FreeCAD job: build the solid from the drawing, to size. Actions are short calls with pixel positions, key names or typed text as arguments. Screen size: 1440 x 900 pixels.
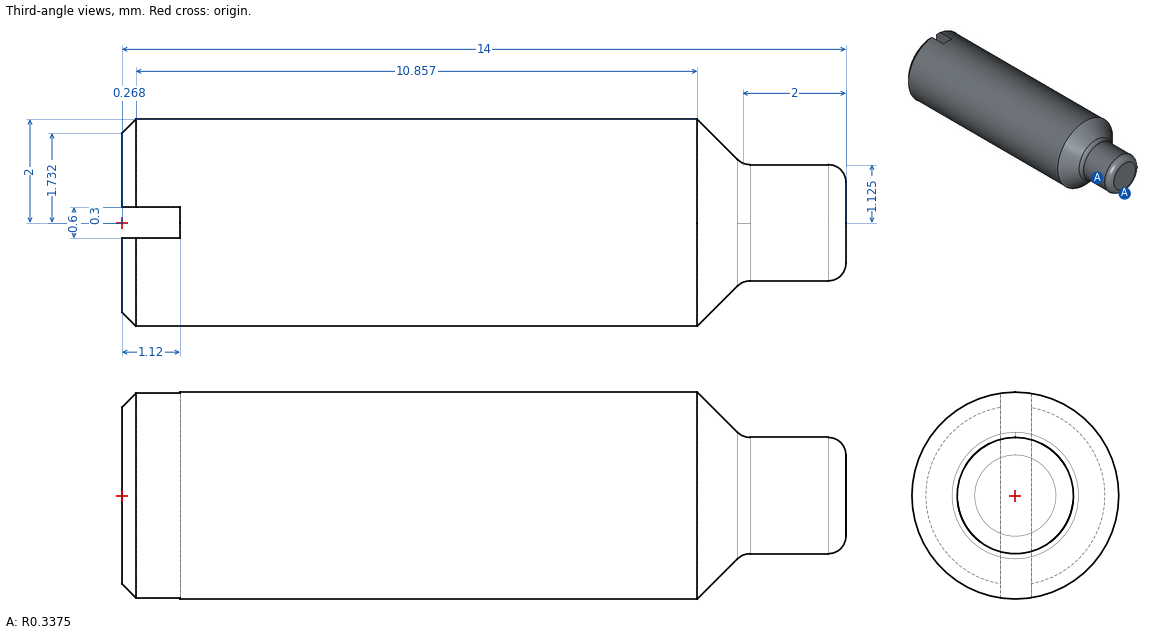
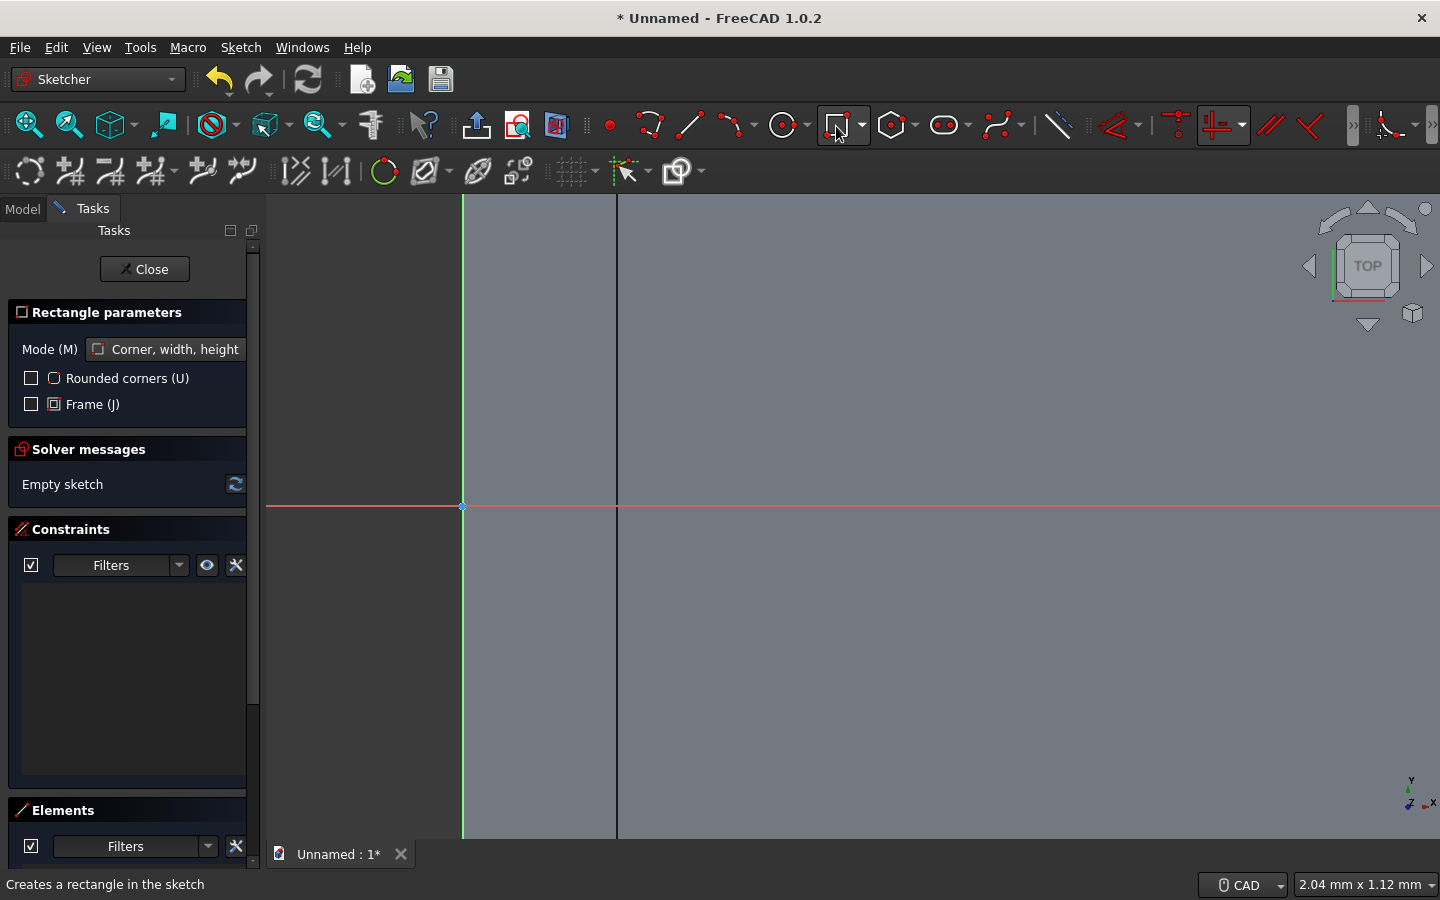
click(463, 334)
click(1107, 679)
key(Escape)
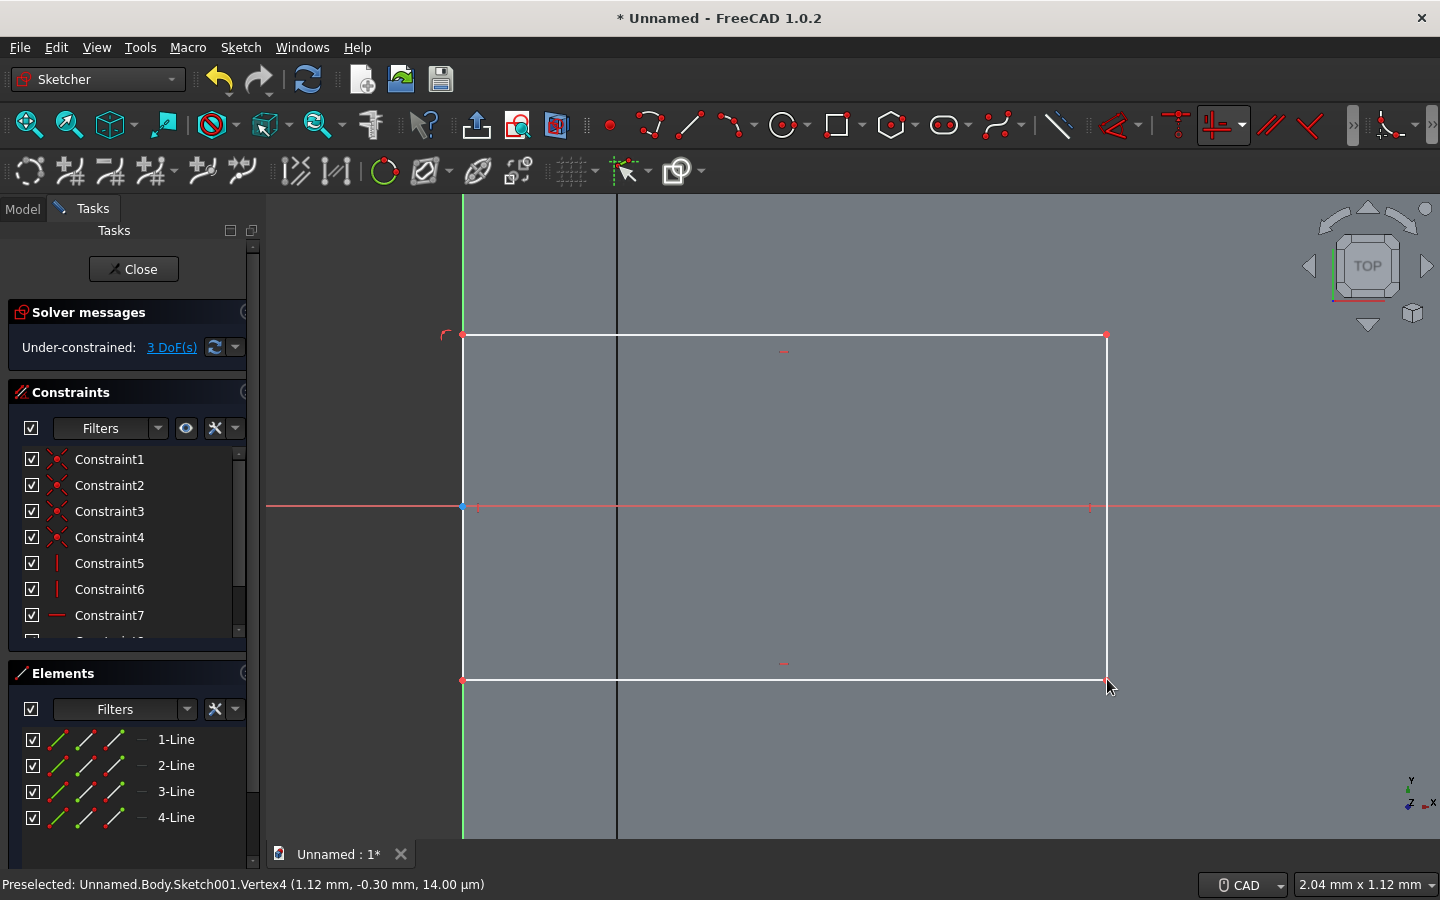
key(d)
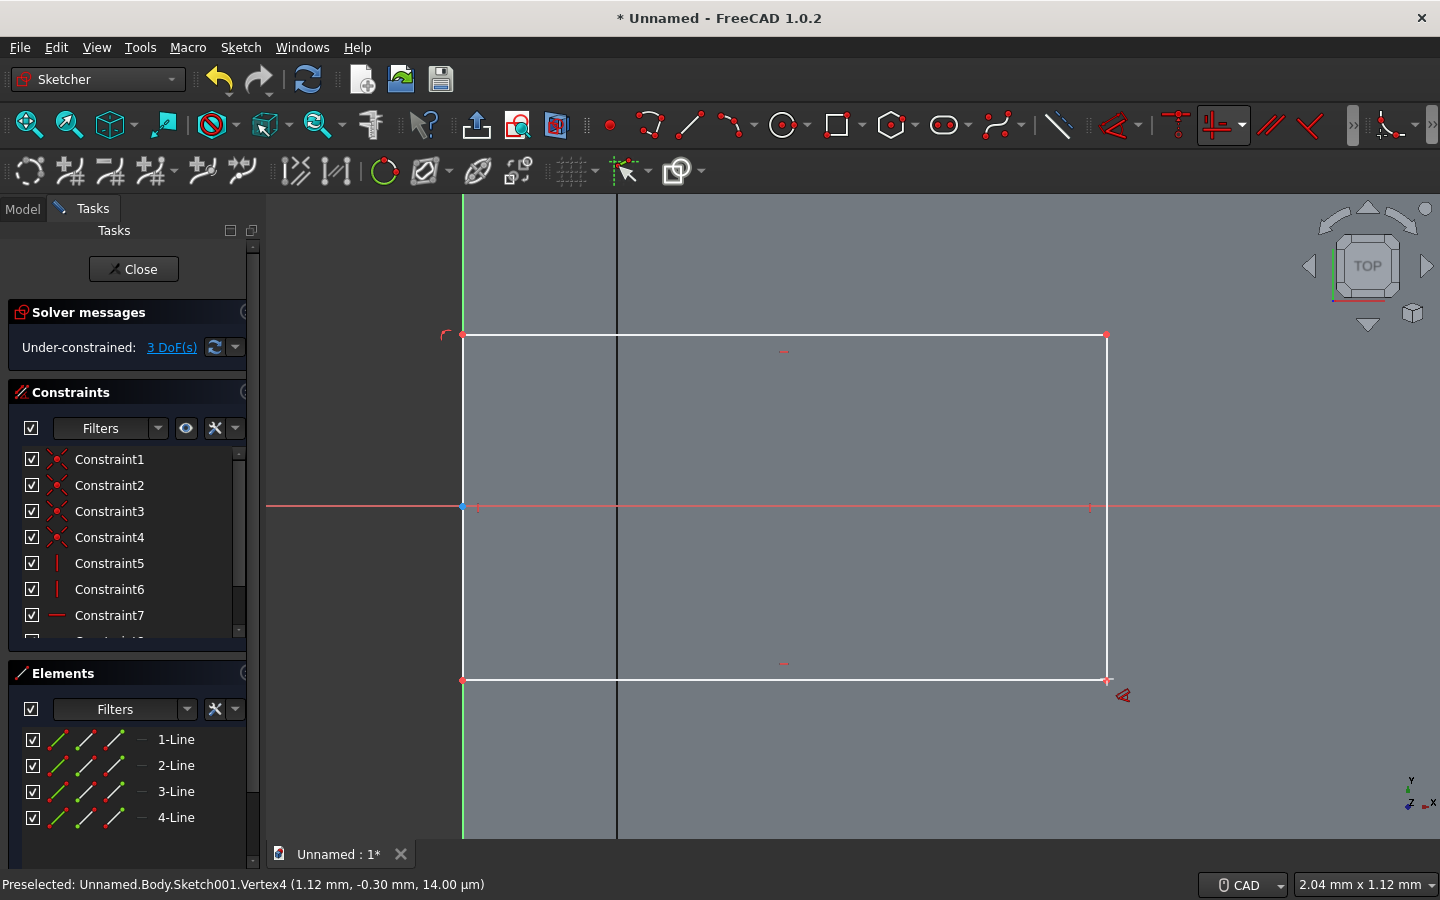
click(463, 438)
click(429, 428)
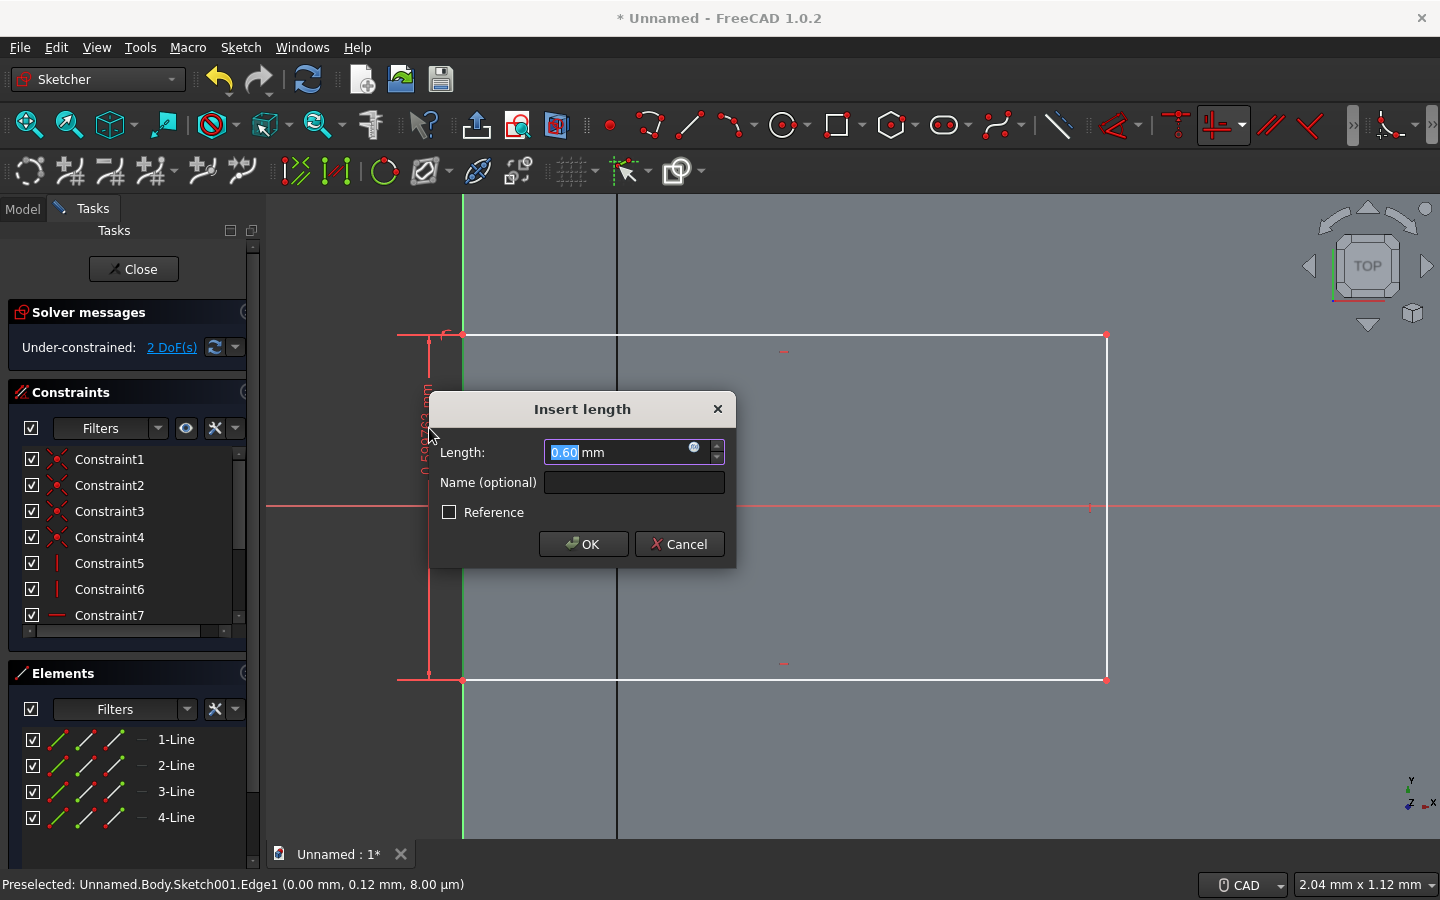
text(0.6)
key(Return)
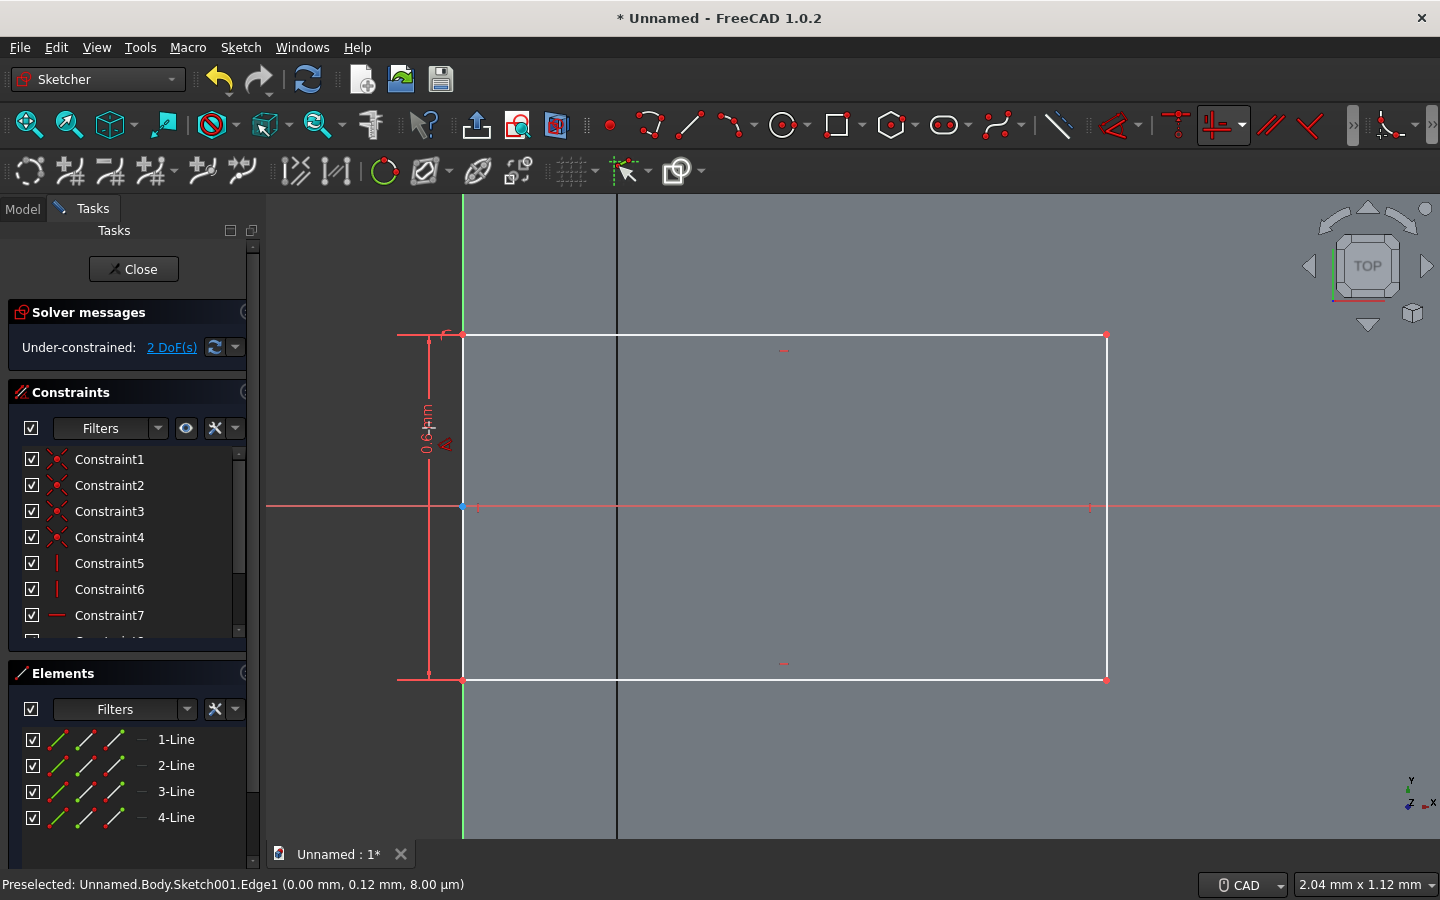
click(656, 680)
click(785, 714)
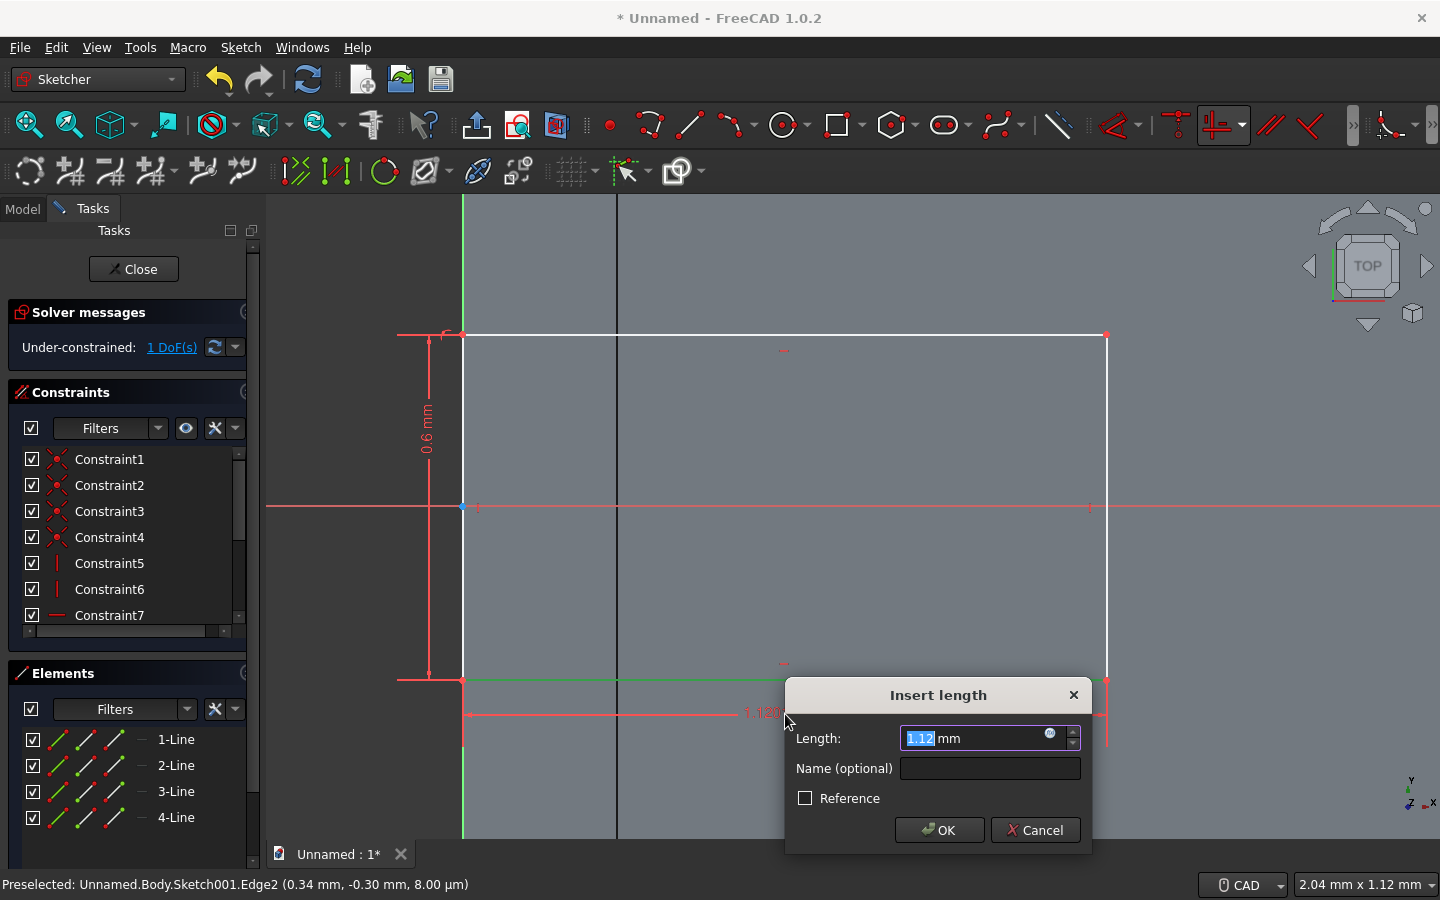
text(1.12)
key(Return)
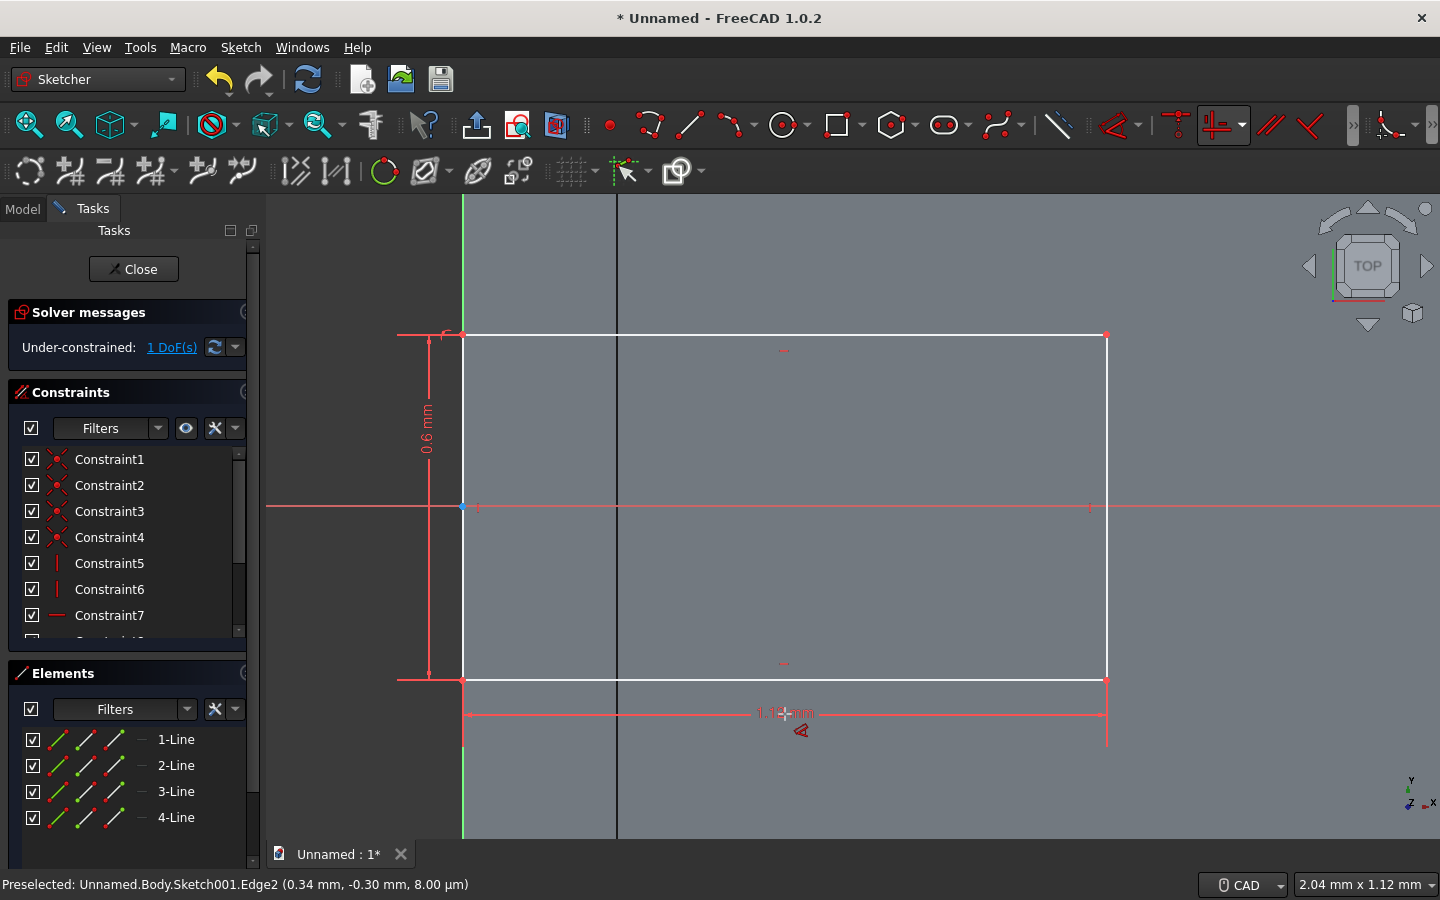
click(463, 335)
click(429, 381)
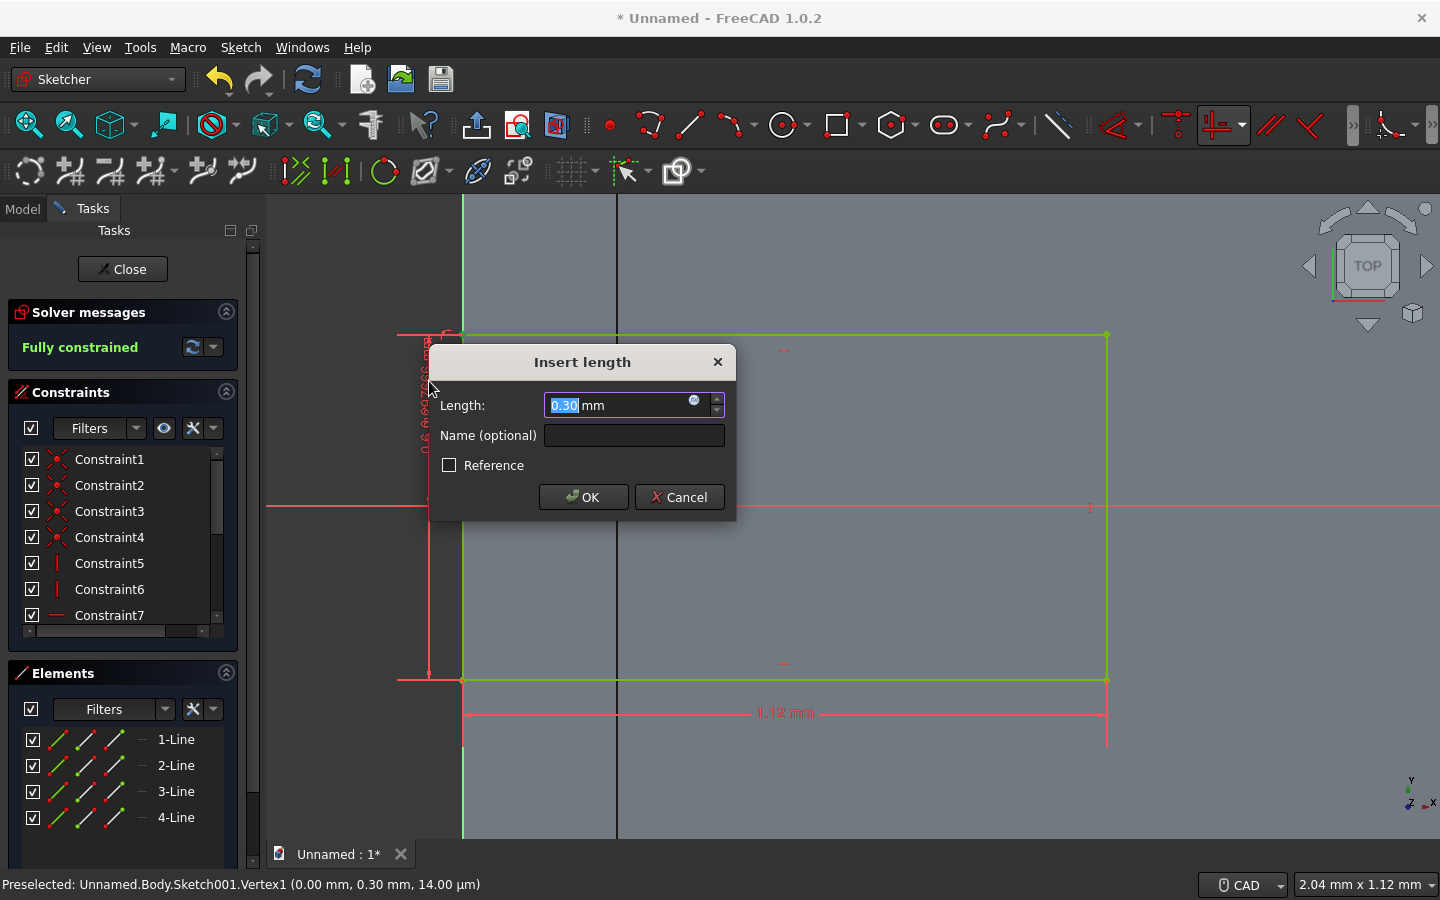
text(0.3)
key(Return)
key(Escape)